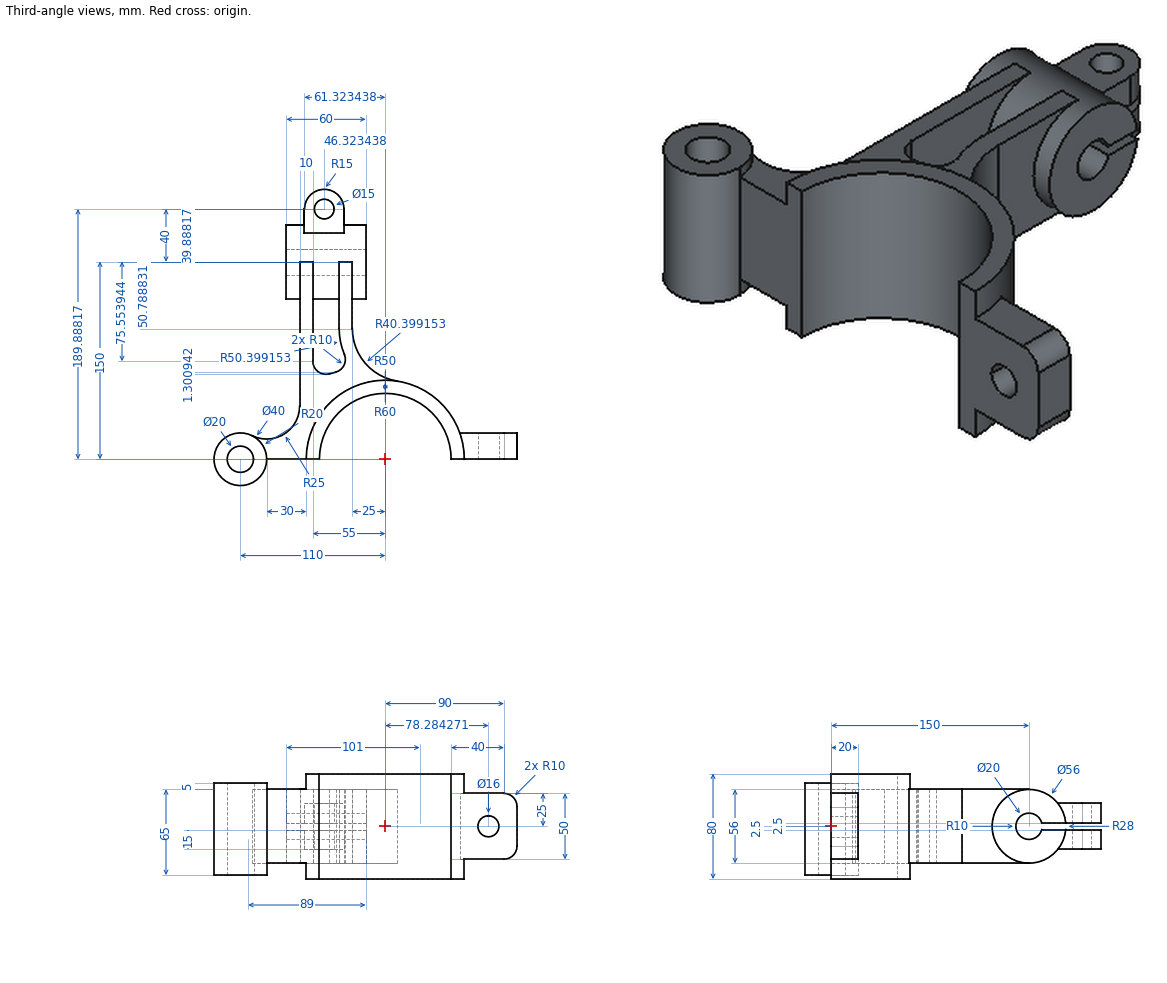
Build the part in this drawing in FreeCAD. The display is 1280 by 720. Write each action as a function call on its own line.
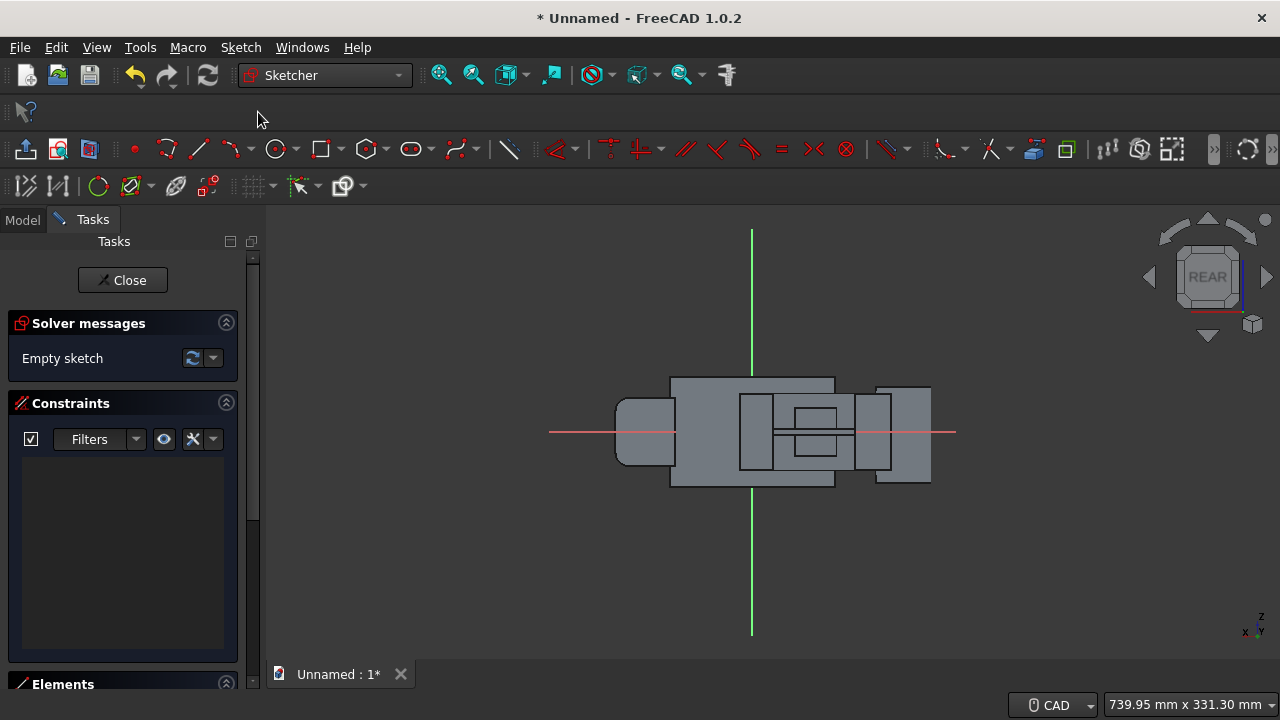
scroll(640, 432, up, 13)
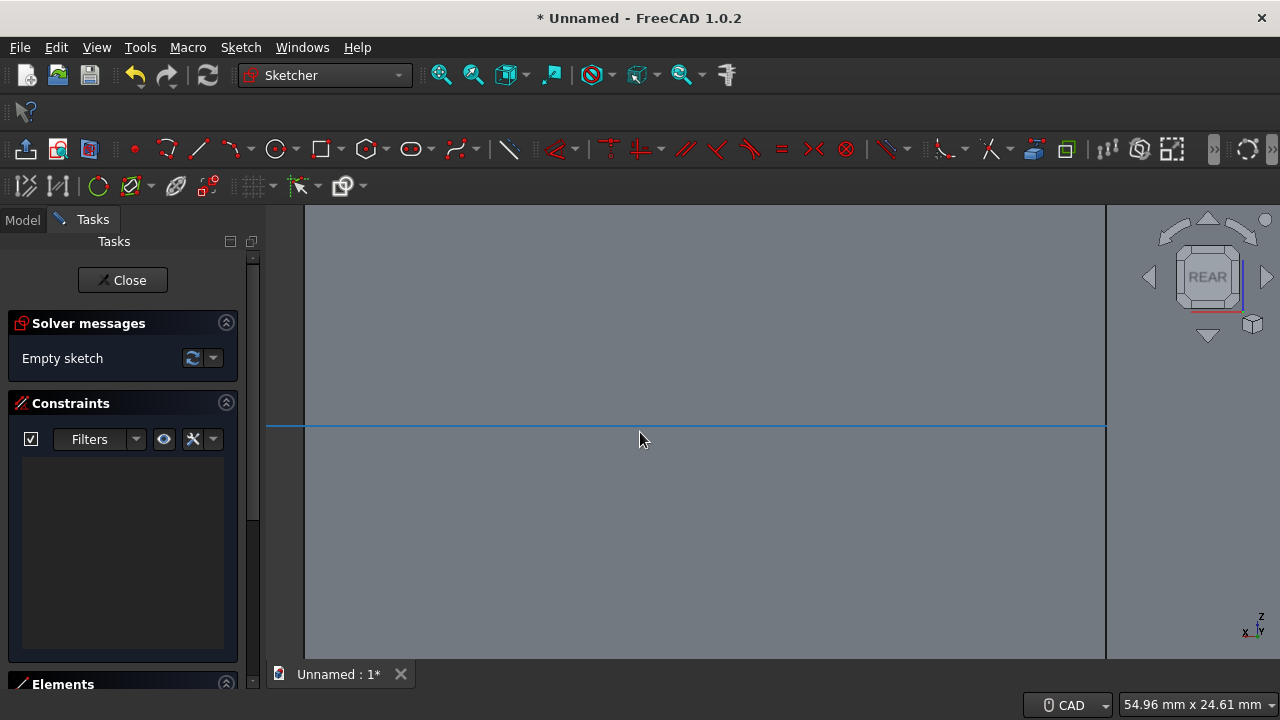
key(g)
key(c)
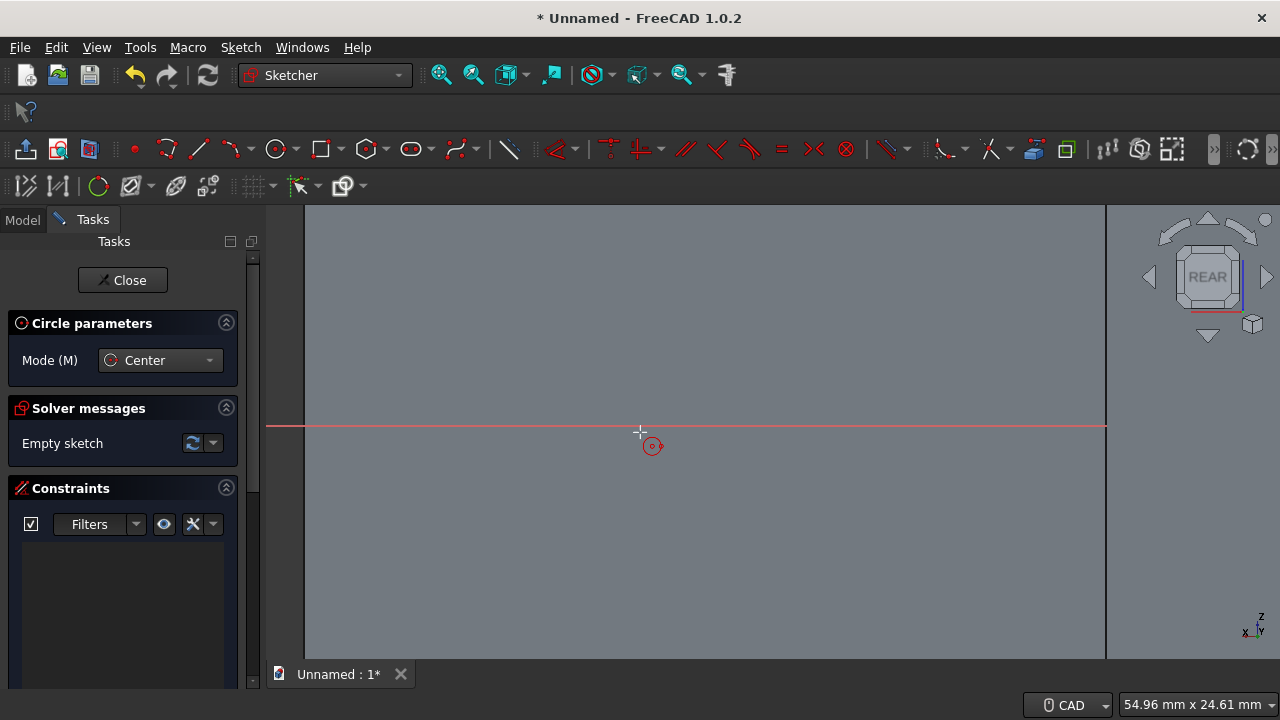
click(705, 426)
move(809, 321)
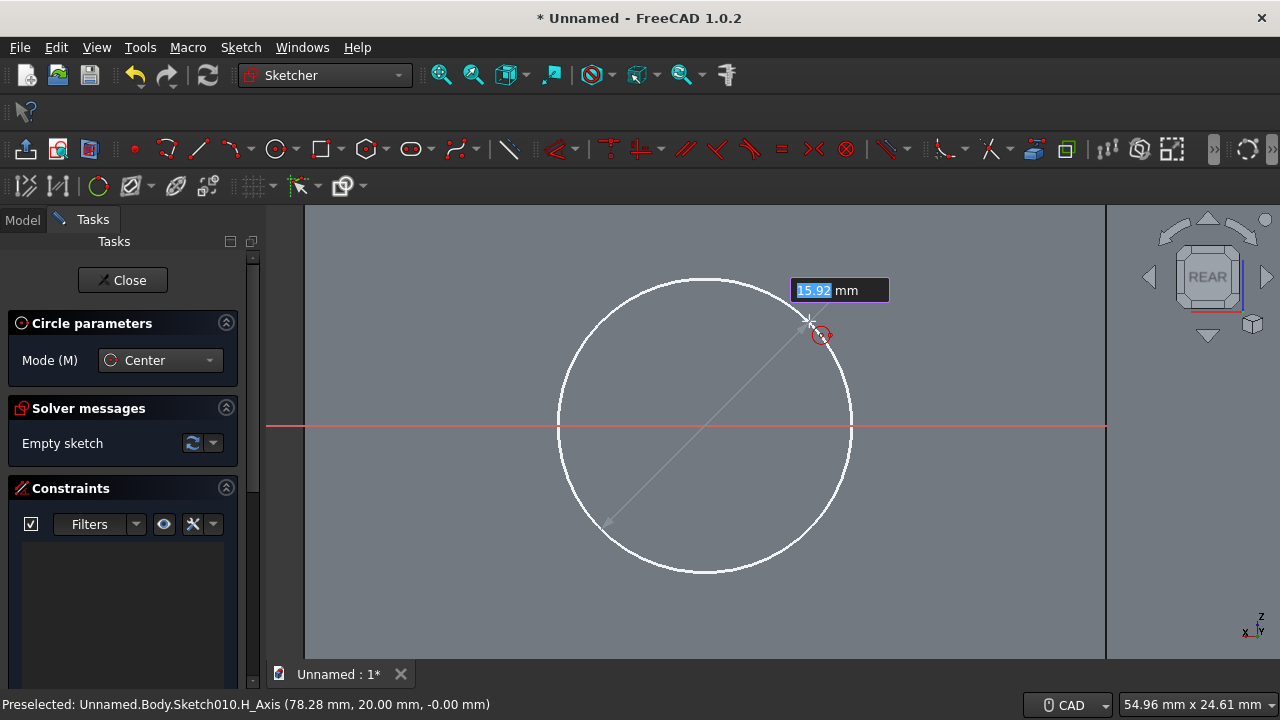
text(16)
key(Return)
key(Escape)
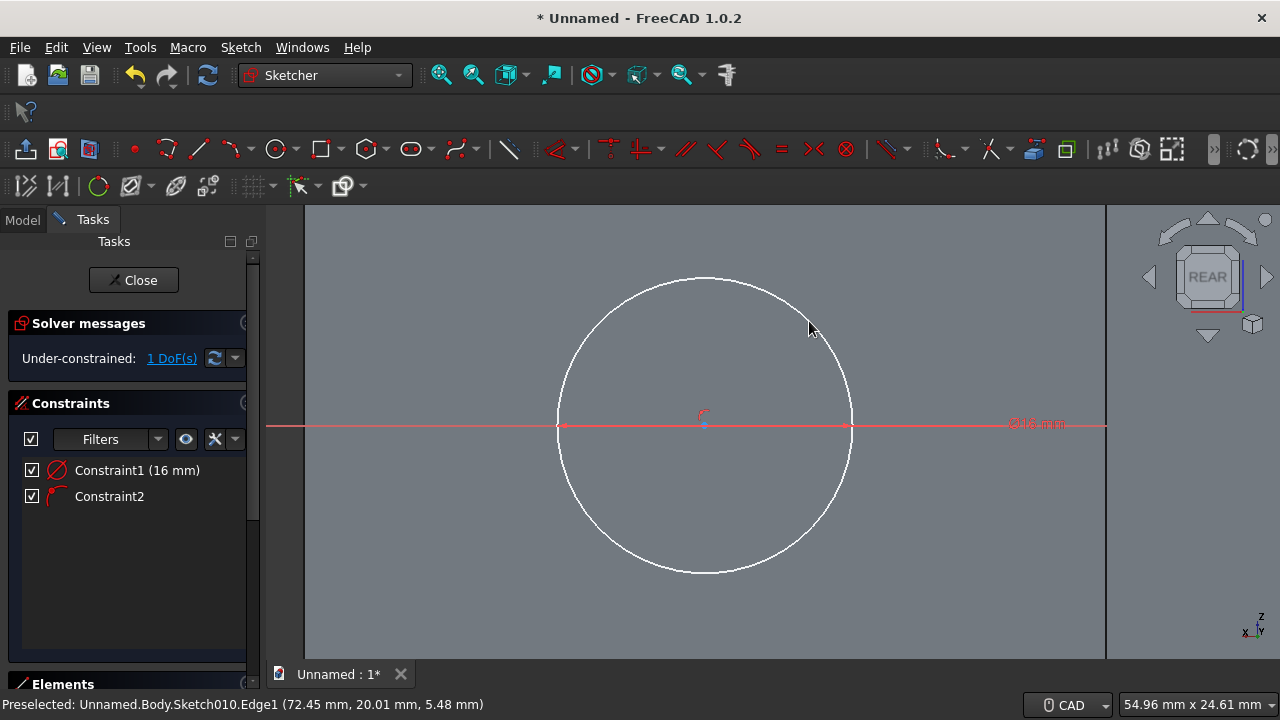
click(556, 150)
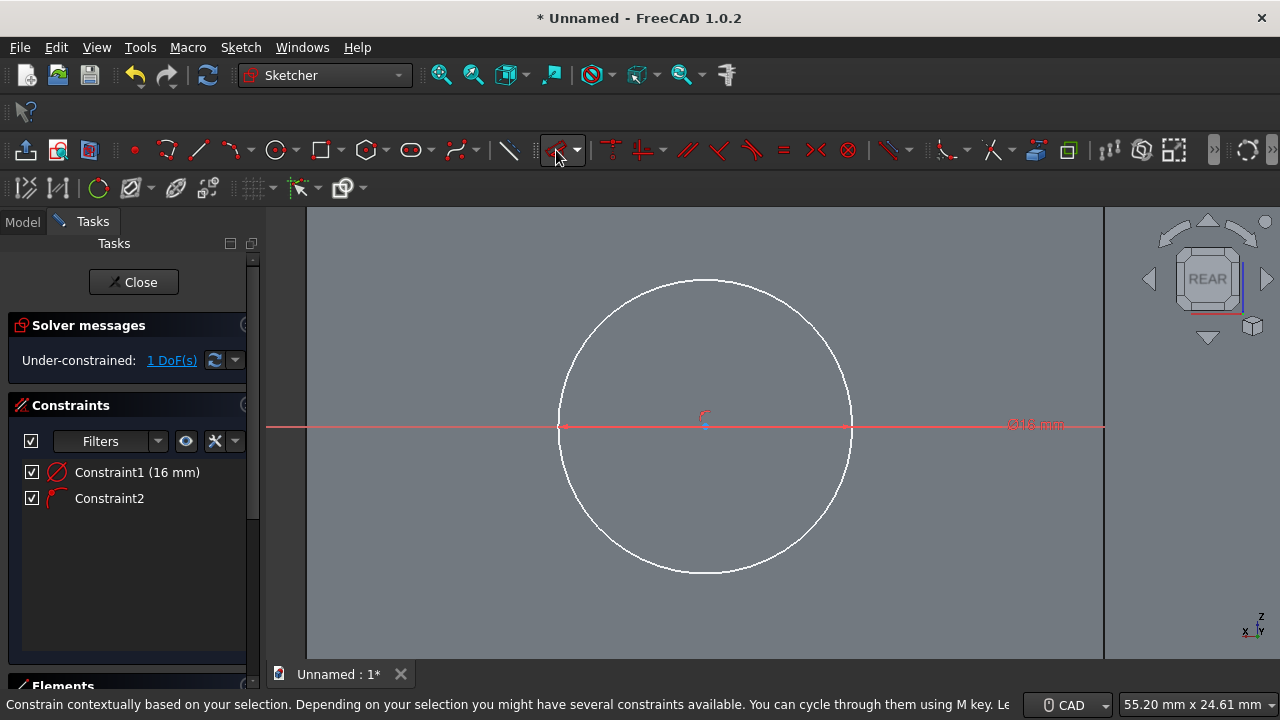
click(705, 427)
click(910, 461)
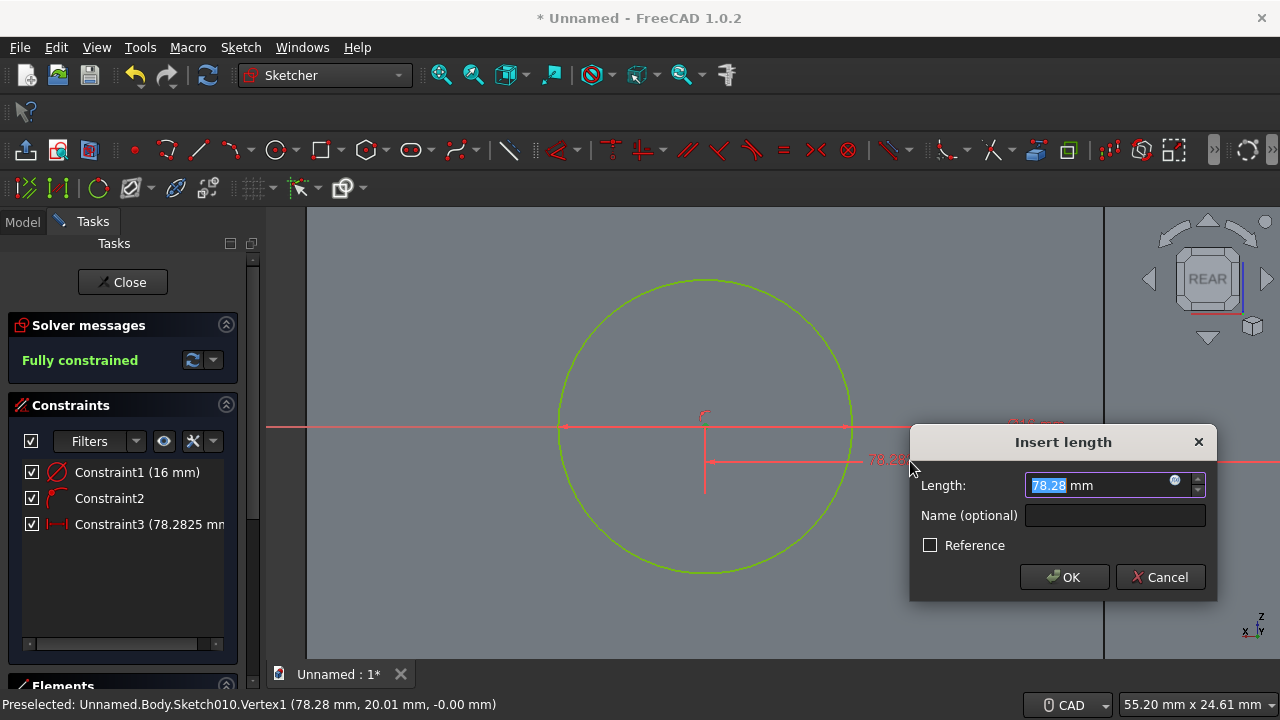
text(78.284271)
key(Return)
key(Escape)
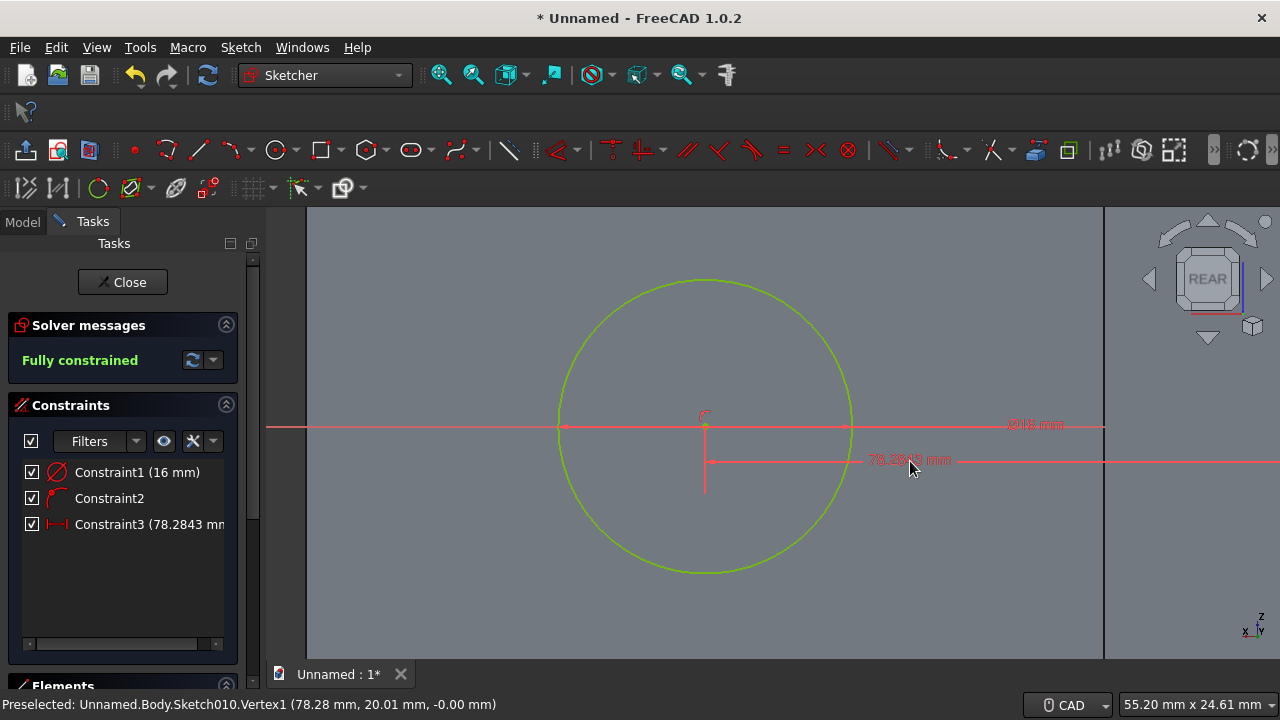
click(123, 282)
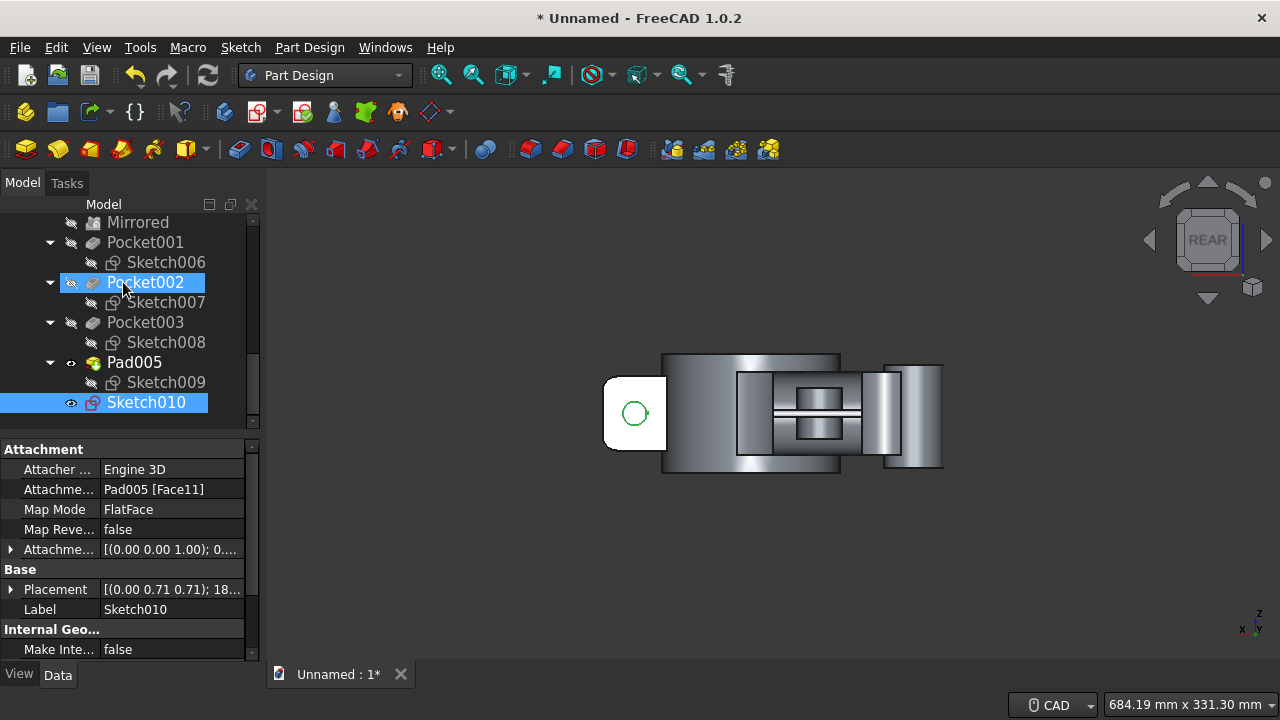
click(240, 150)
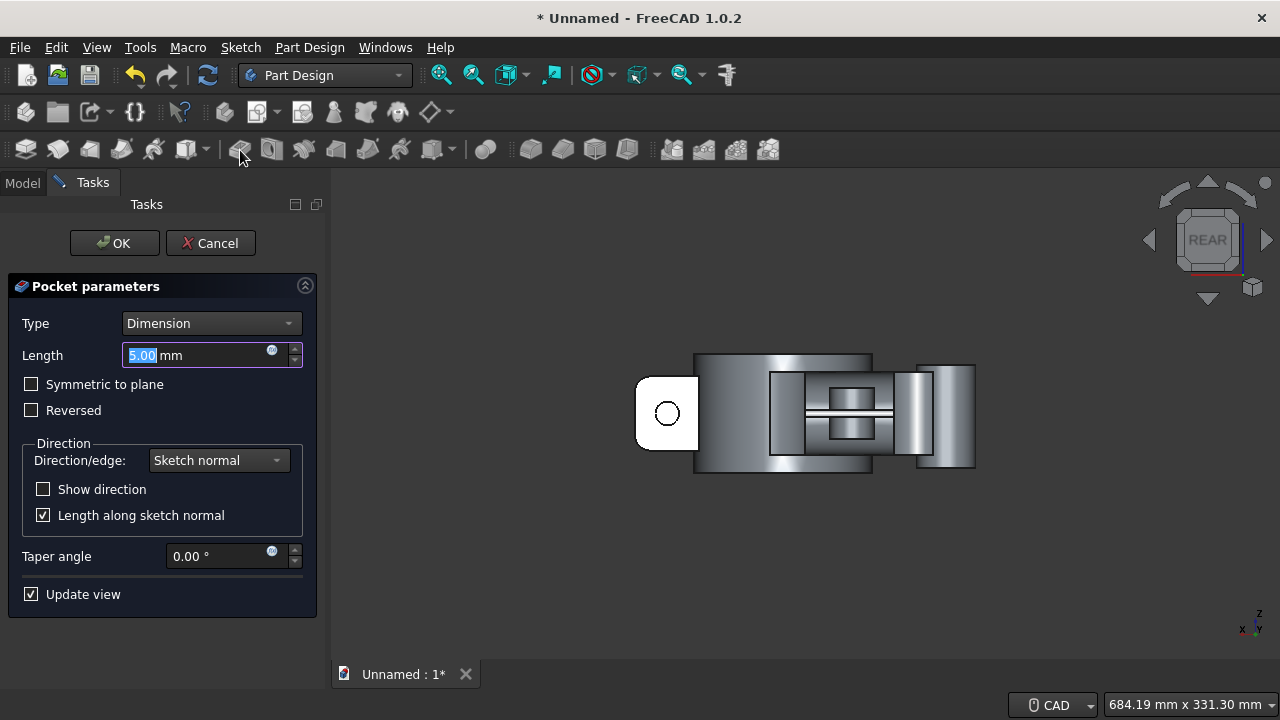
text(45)
key(Tab)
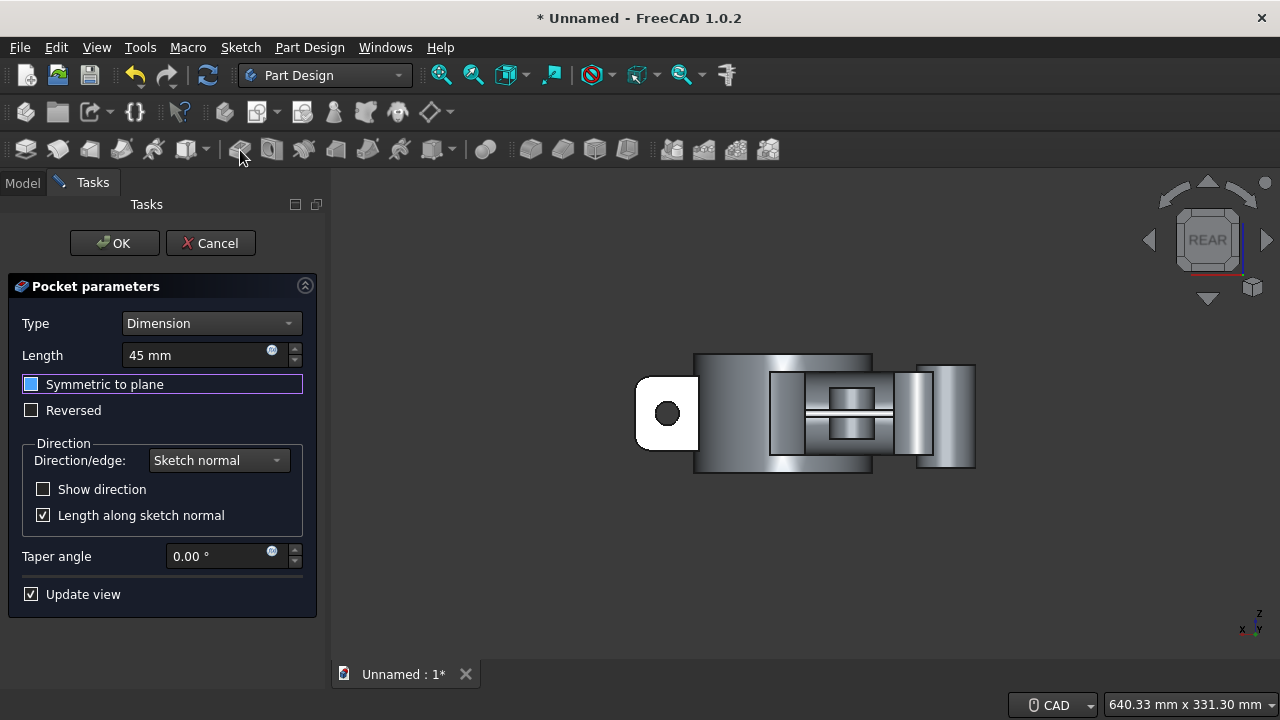
click(115, 243)